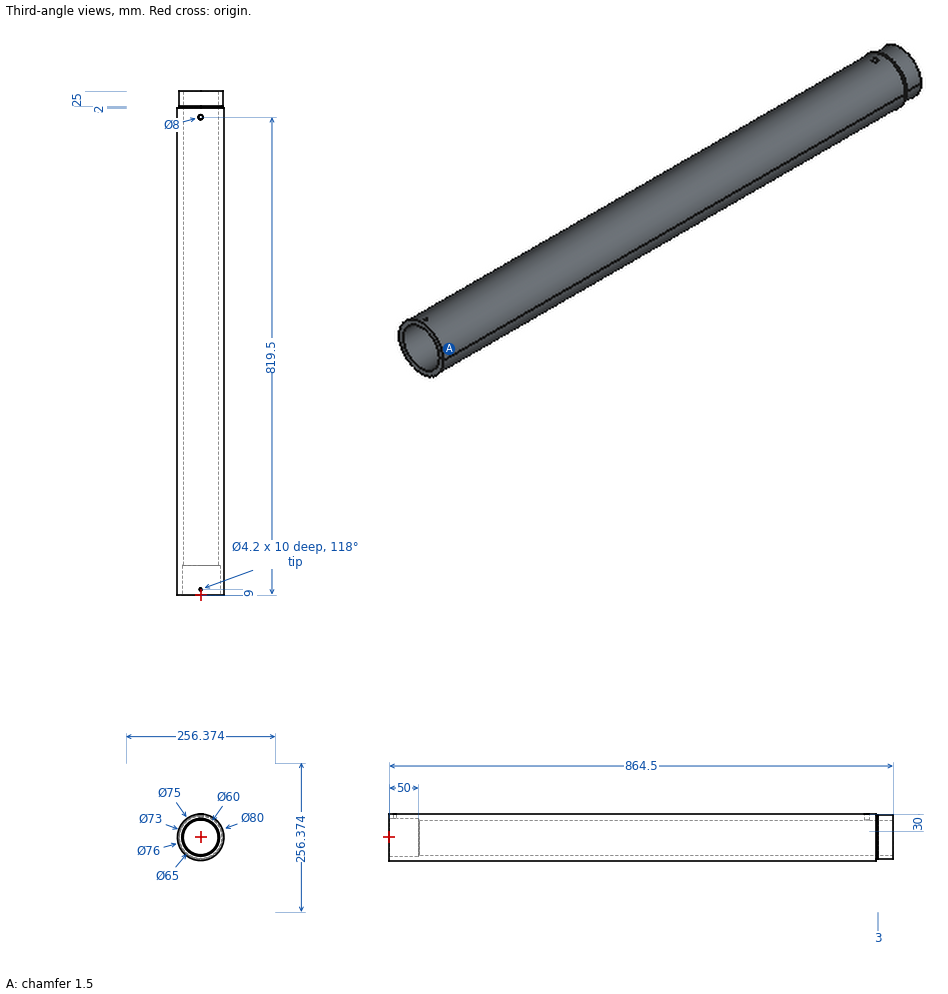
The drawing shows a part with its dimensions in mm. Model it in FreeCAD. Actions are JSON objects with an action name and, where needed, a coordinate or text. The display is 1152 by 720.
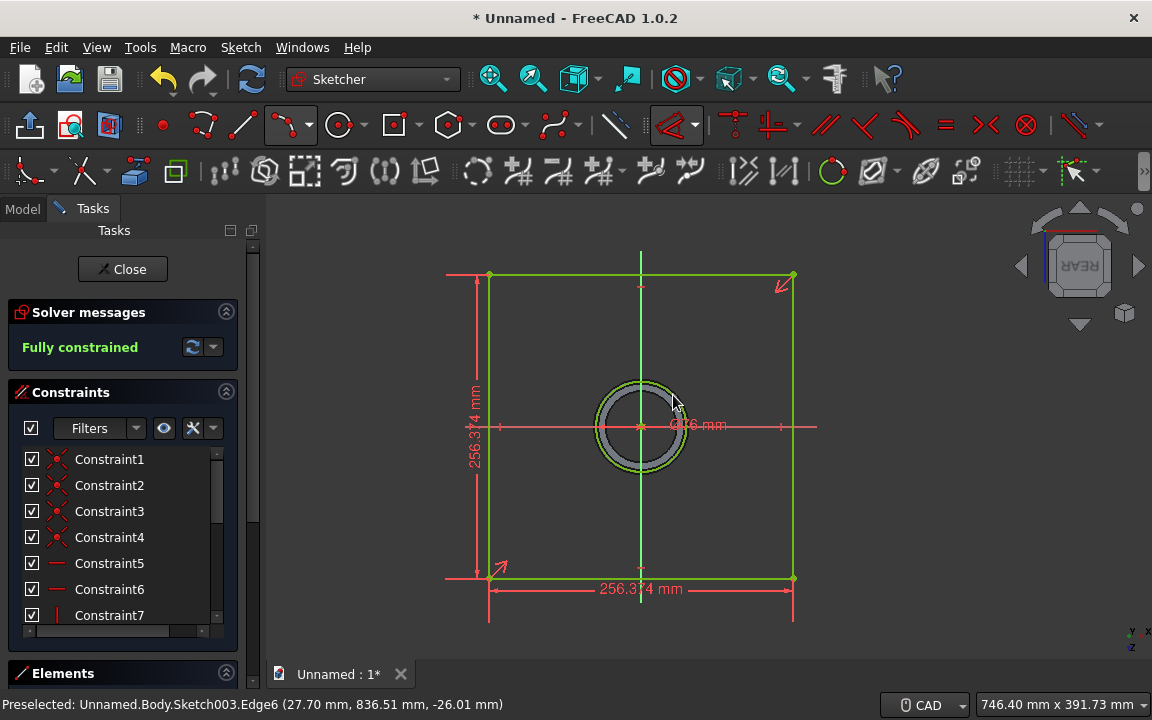
{"action": "left_click", "coordinate": [123, 269]}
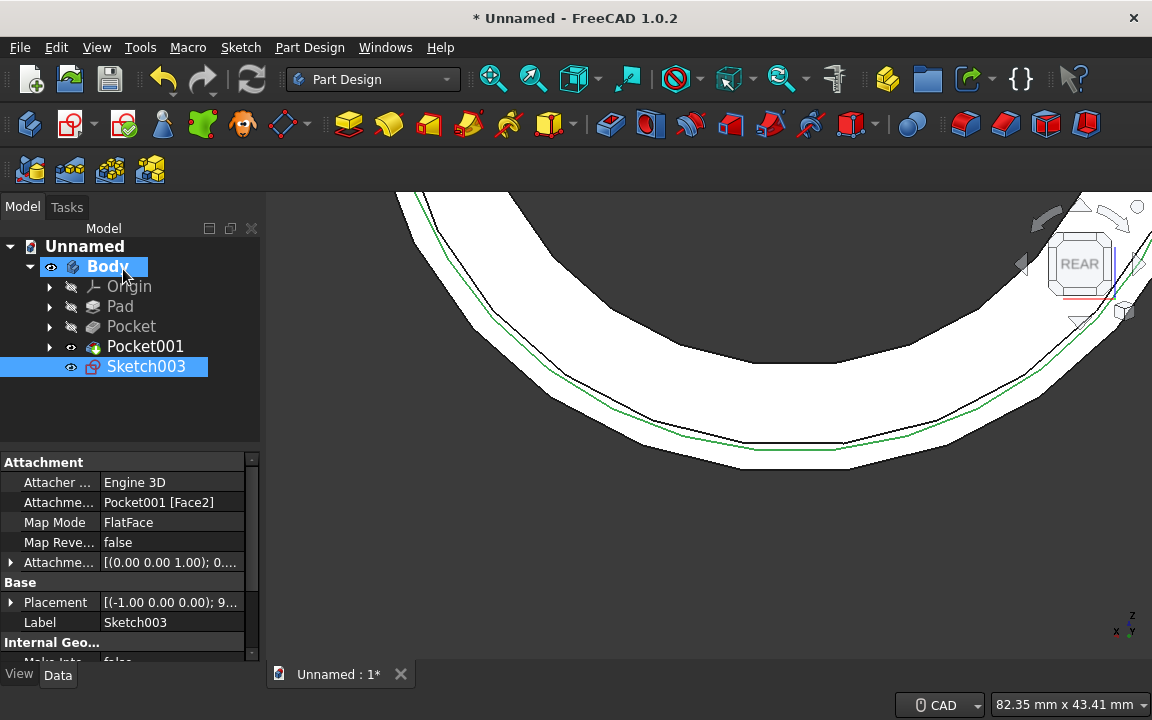
{"action": "left_click", "coordinate": [612, 124]}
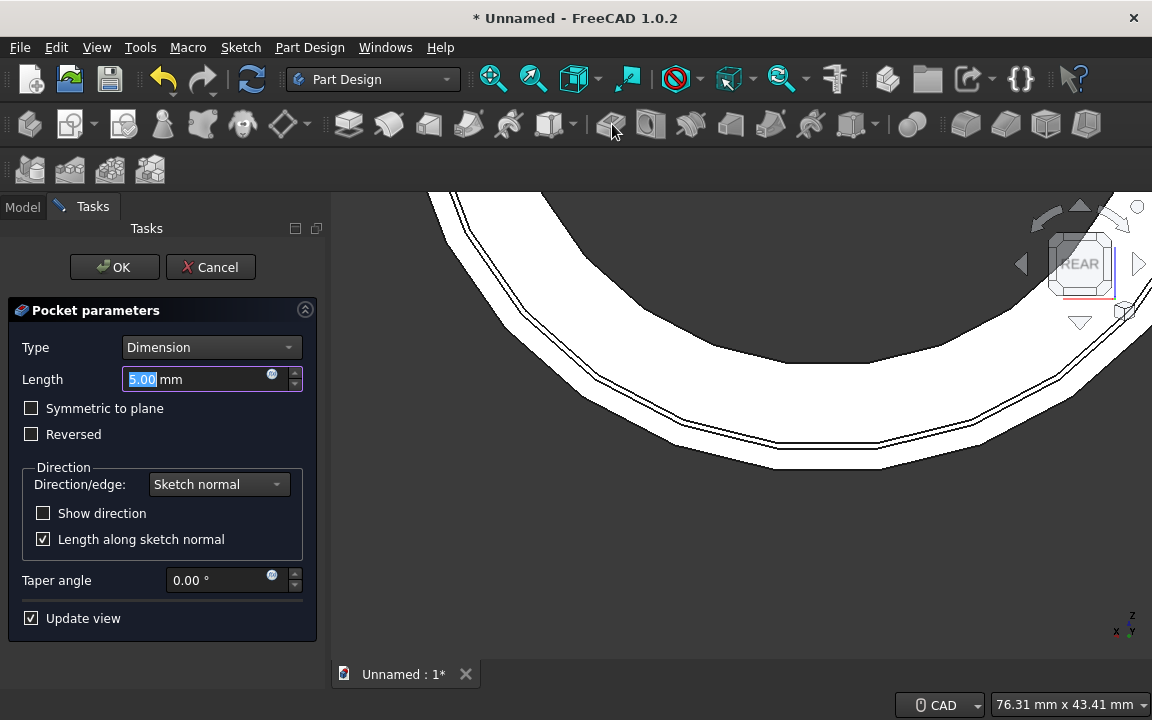
{"action": "type", "text": "2"}
{"action": "key", "text": "Tab"}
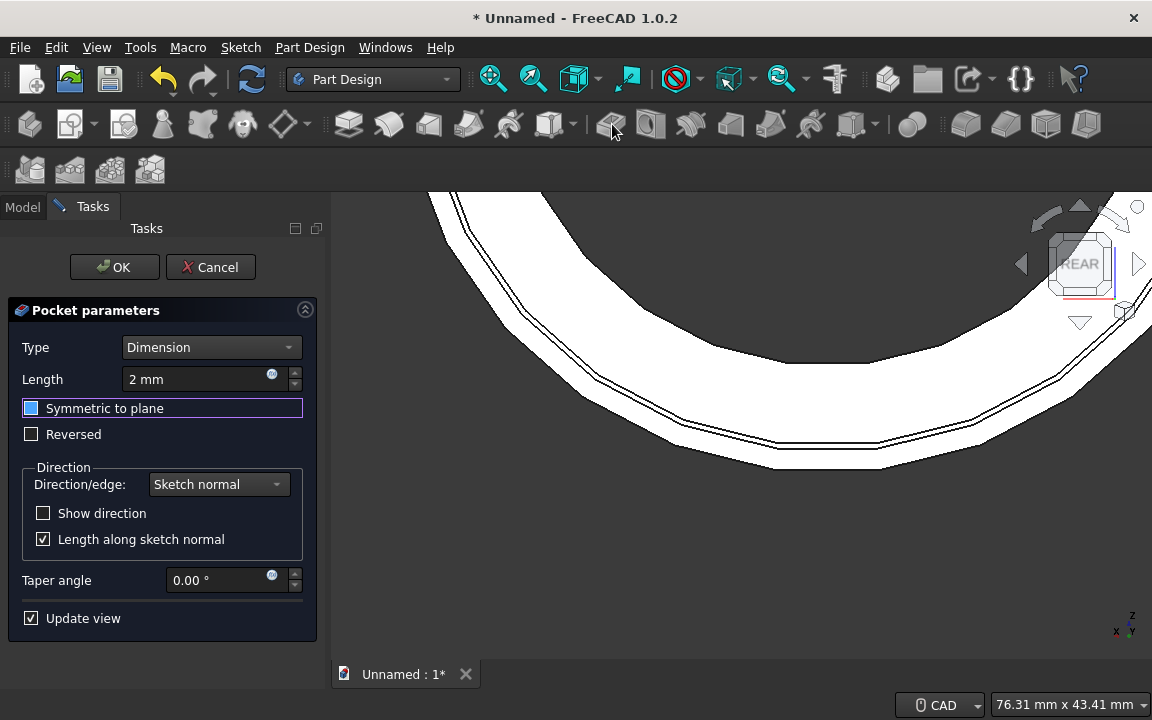
{"action": "left_click", "coordinate": [115, 267]}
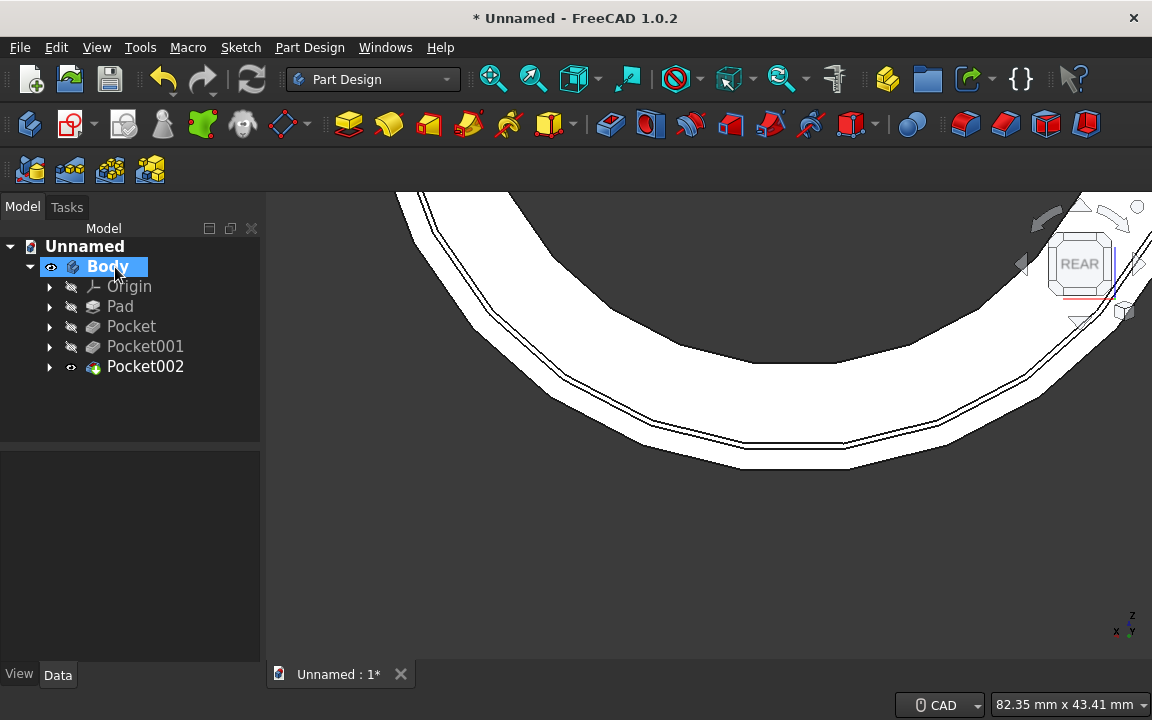
{"action": "left_click", "coordinate": [494, 80]}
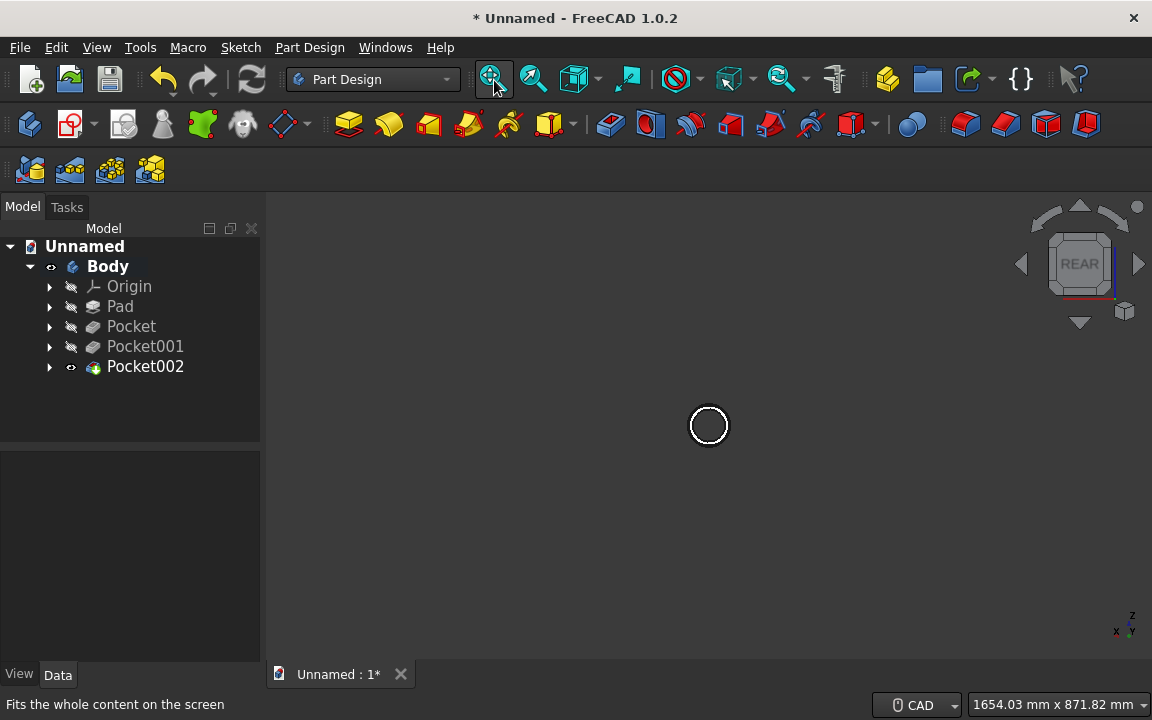
{"action": "left_click", "coordinate": [70, 124]}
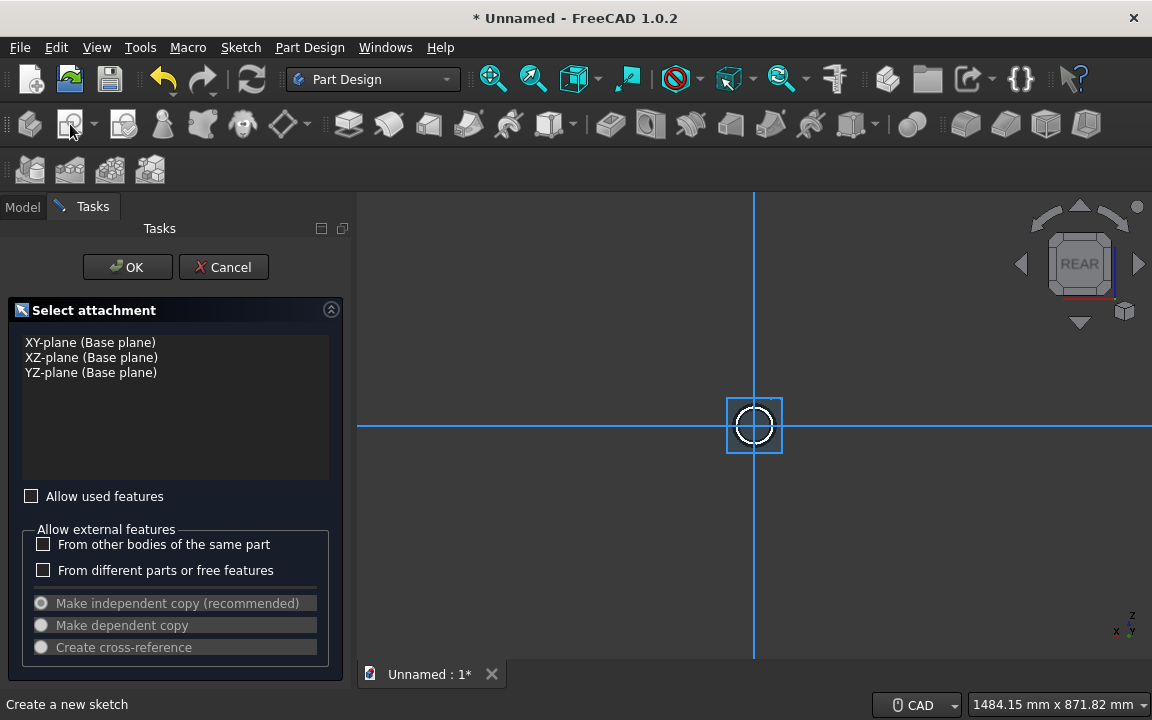
{"action": "left_click", "coordinate": [82, 358]}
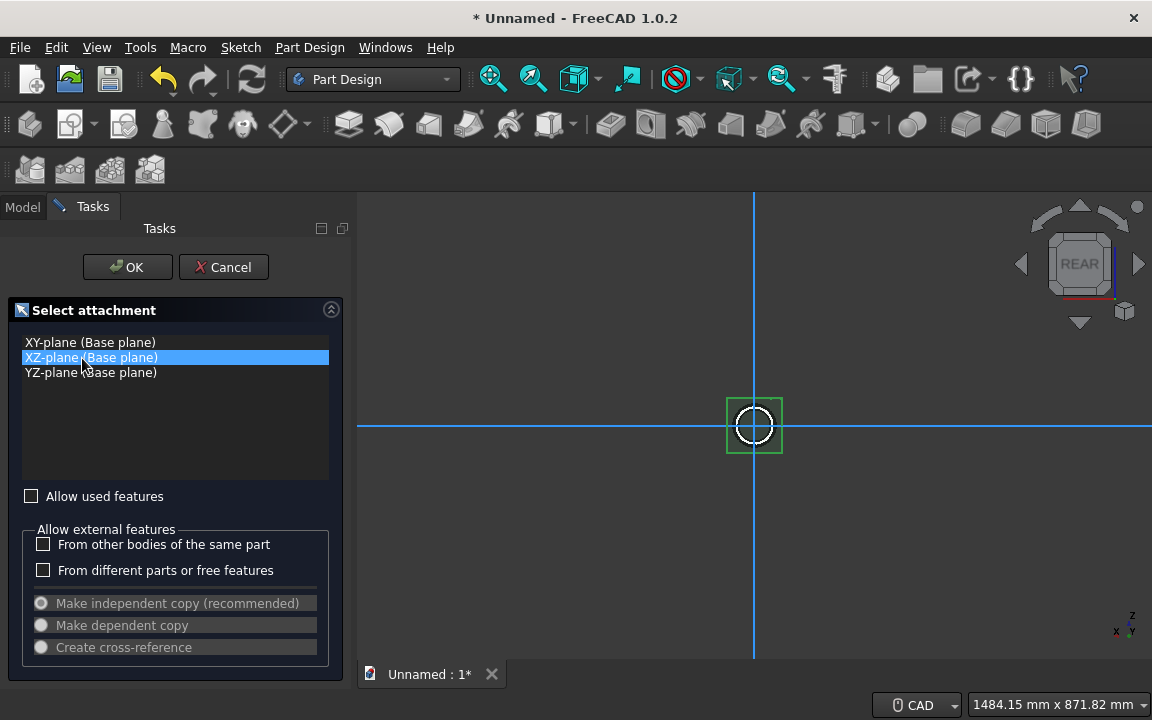
{"action": "left_click", "coordinate": [128, 267]}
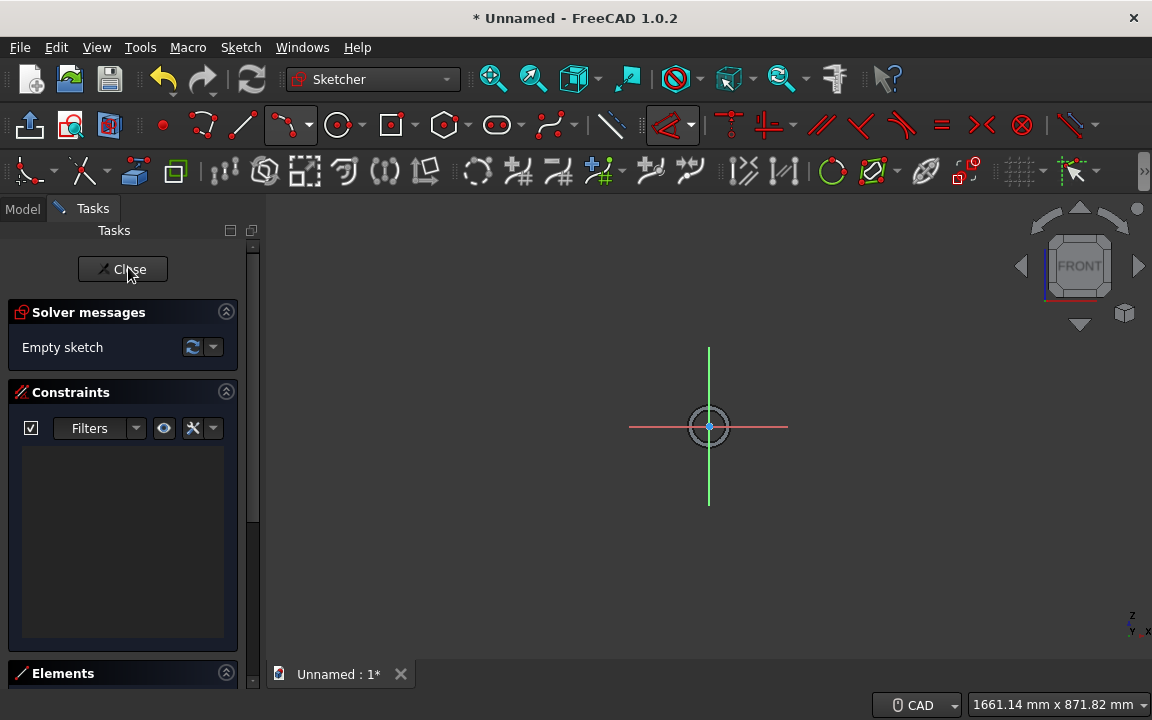
{"action": "scroll", "coordinate": [718, 427], "scroll_direction": "up", "scroll_amount": 11}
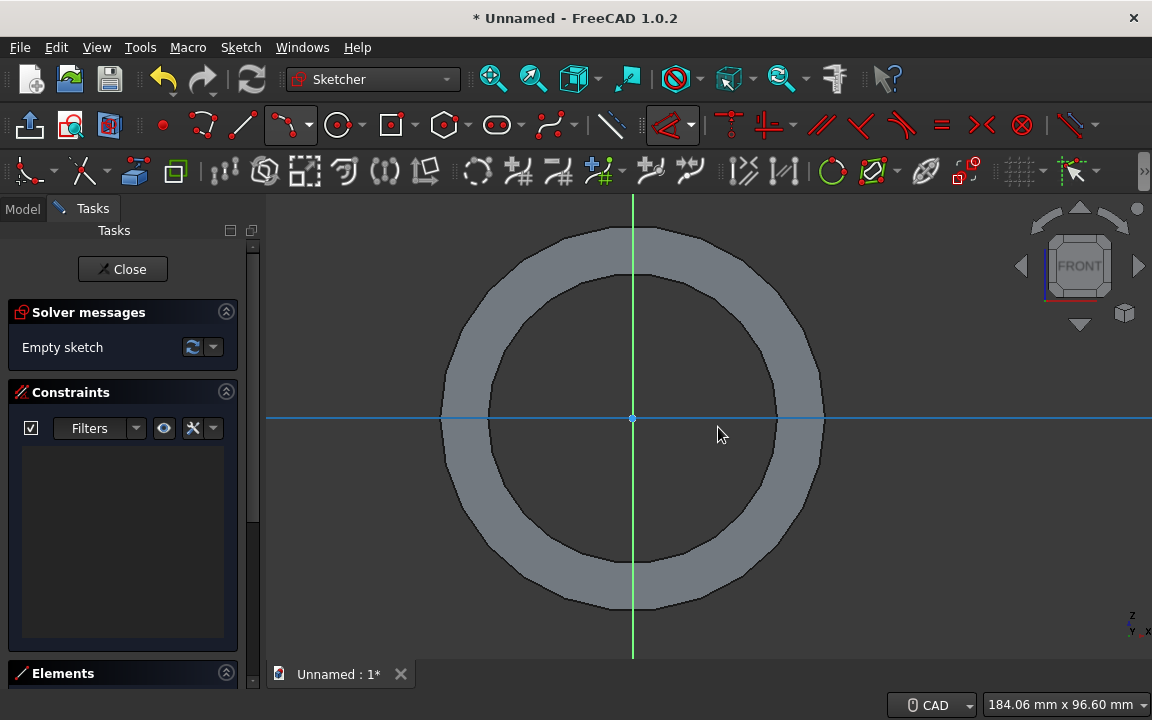
{"action": "key", "text": "g c"}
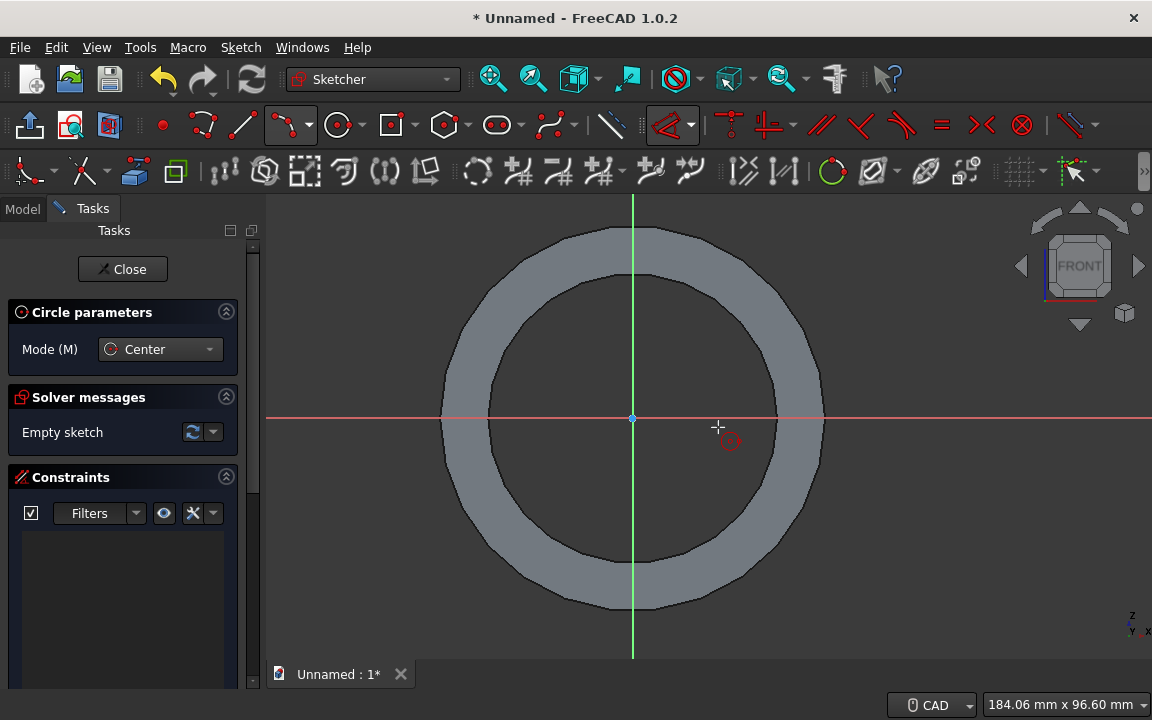
{"action": "left_click", "coordinate": [633, 418]}
{"action": "mouse_move", "coordinate": [743, 308]}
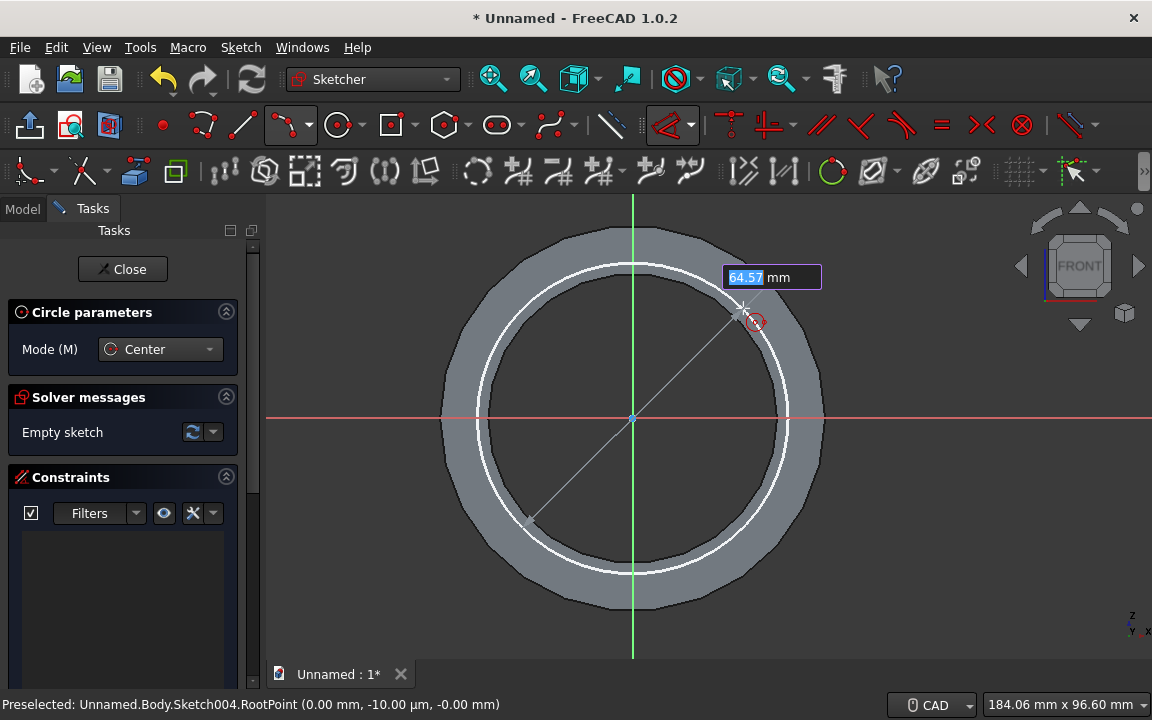
{"action": "type", "text": "65"}
{"action": "key", "text": "Return"}
{"action": "key", "text": "Escape"}